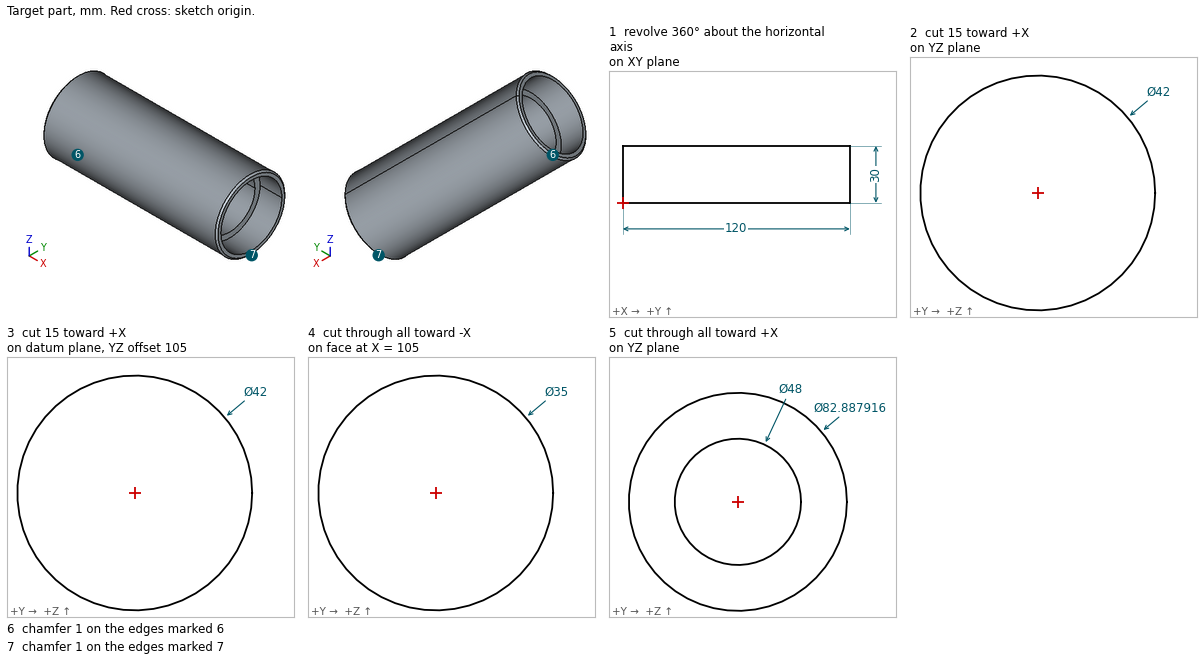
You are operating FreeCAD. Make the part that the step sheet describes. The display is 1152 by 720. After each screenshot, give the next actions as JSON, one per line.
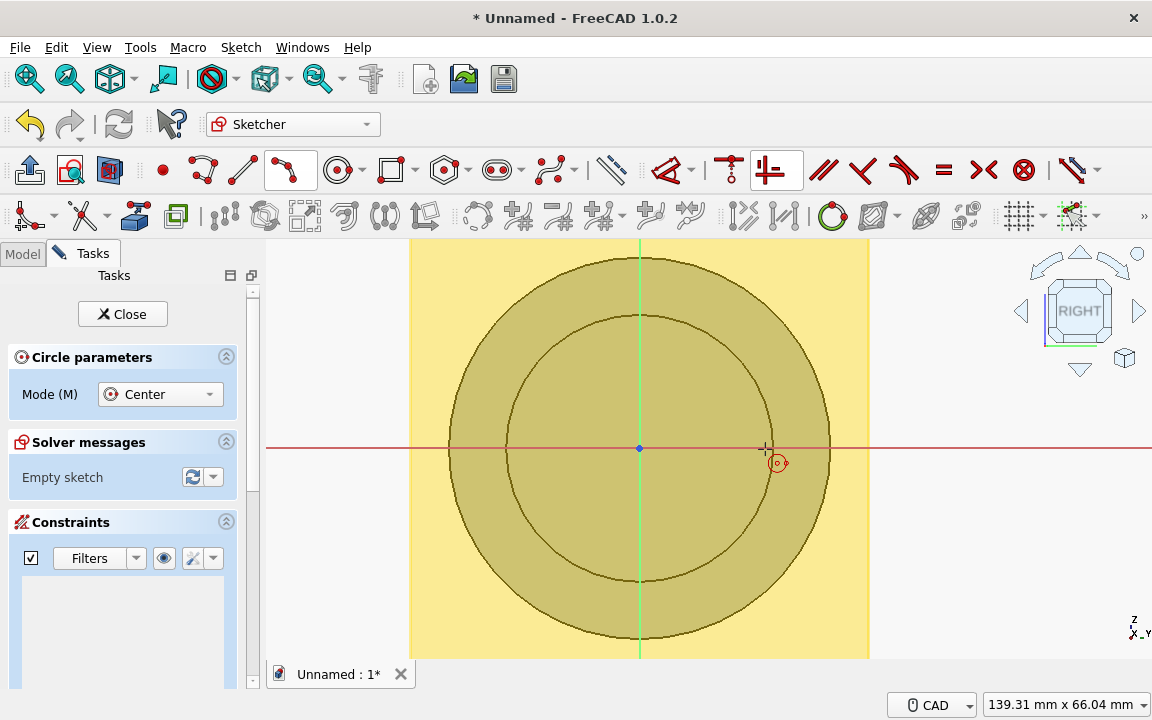
{"action": "left_click", "coordinate": [640, 448]}
{"action": "left_click", "coordinate": [734, 354]}
{"action": "key", "text": "Escape"}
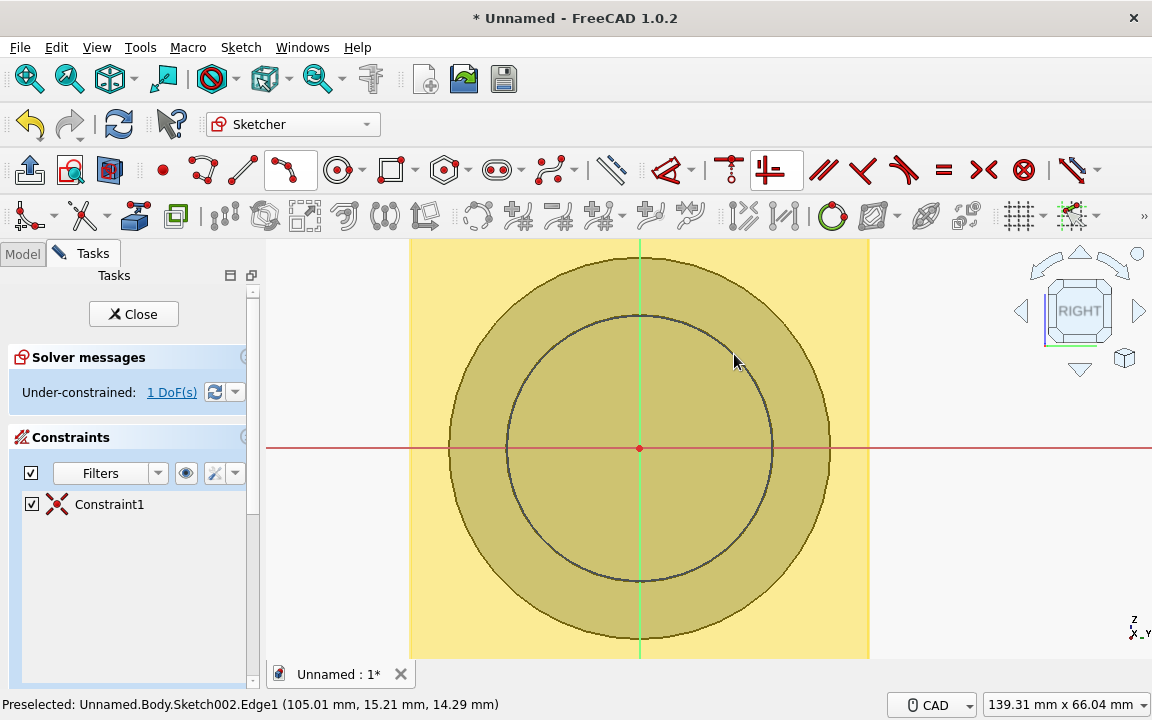
{"action": "key", "text": "d"}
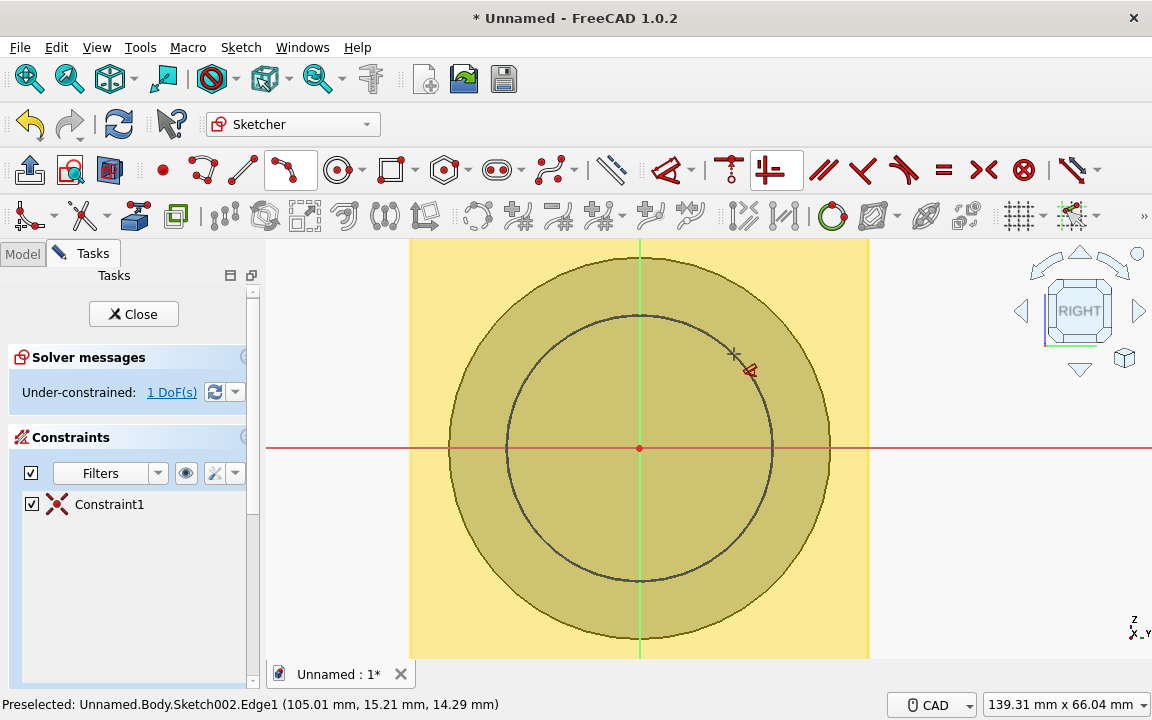
{"action": "left_click", "coordinate": [733, 354]}
{"action": "left_click", "coordinate": [755, 331]}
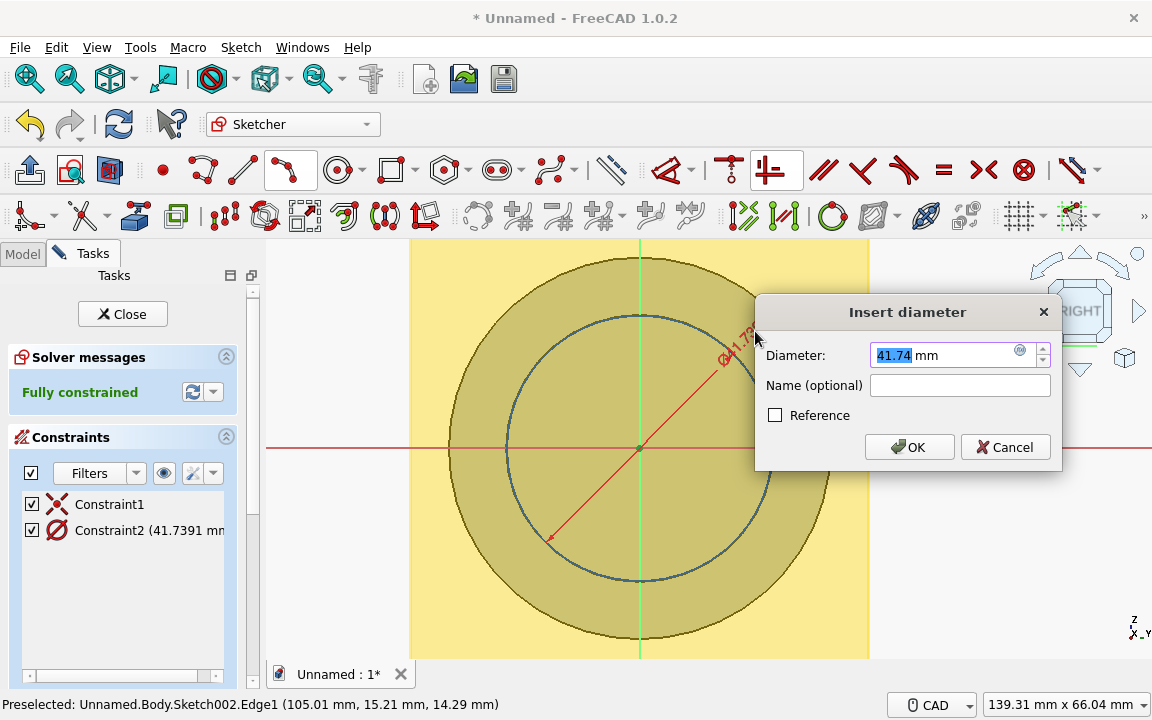
{"action": "type", "text": "42"}
{"action": "key", "text": "Return"}
{"action": "key", "text": "Escape"}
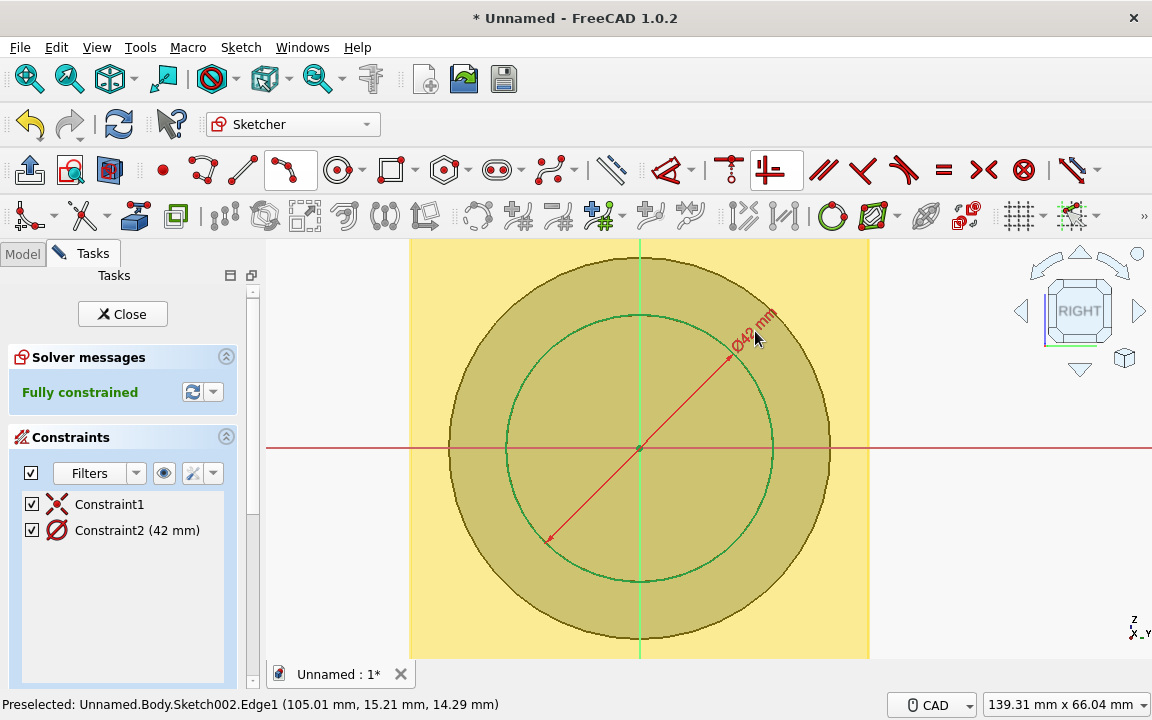
{"action": "left_click", "coordinate": [123, 314]}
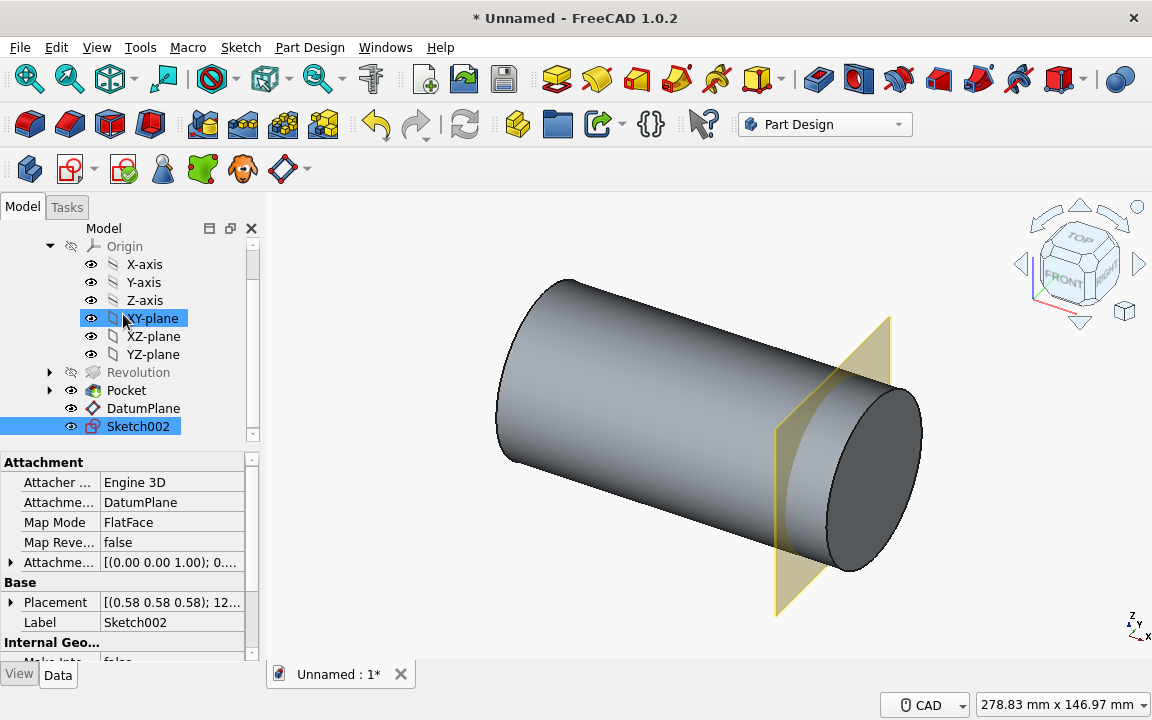
{"action": "left_click", "coordinate": [820, 80]}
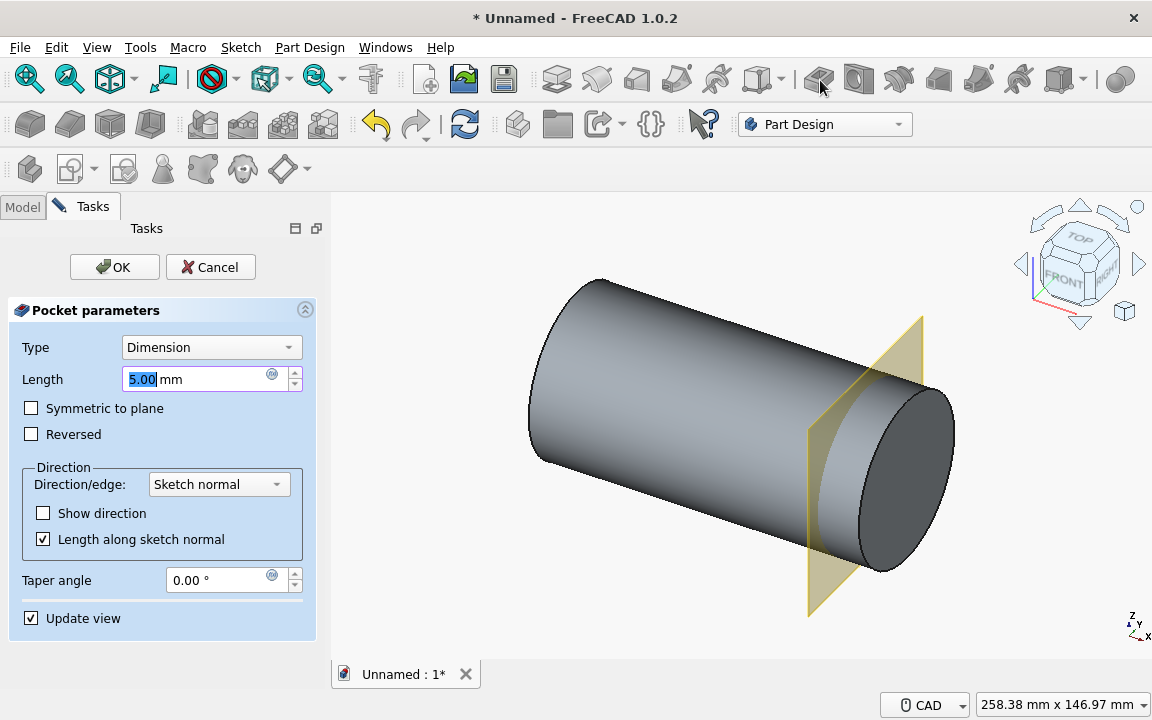
{"action": "type", "text": "15"}
{"action": "key", "text": "Tab"}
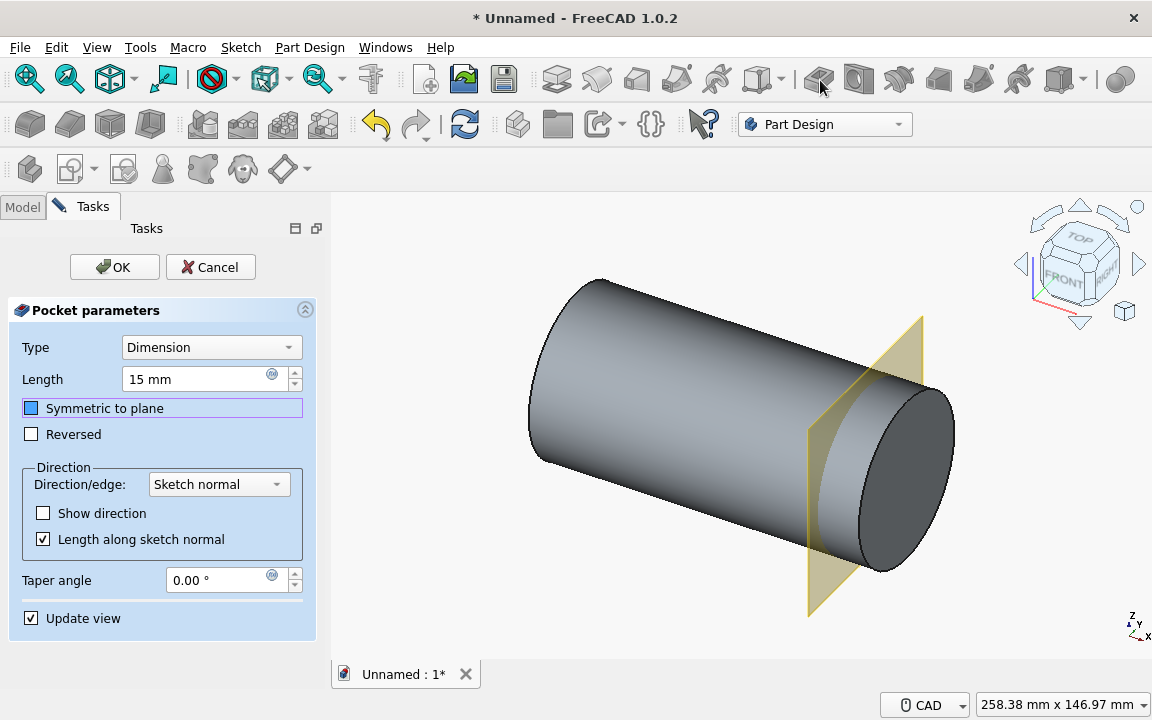
{"action": "left_click", "coordinate": [30, 434]}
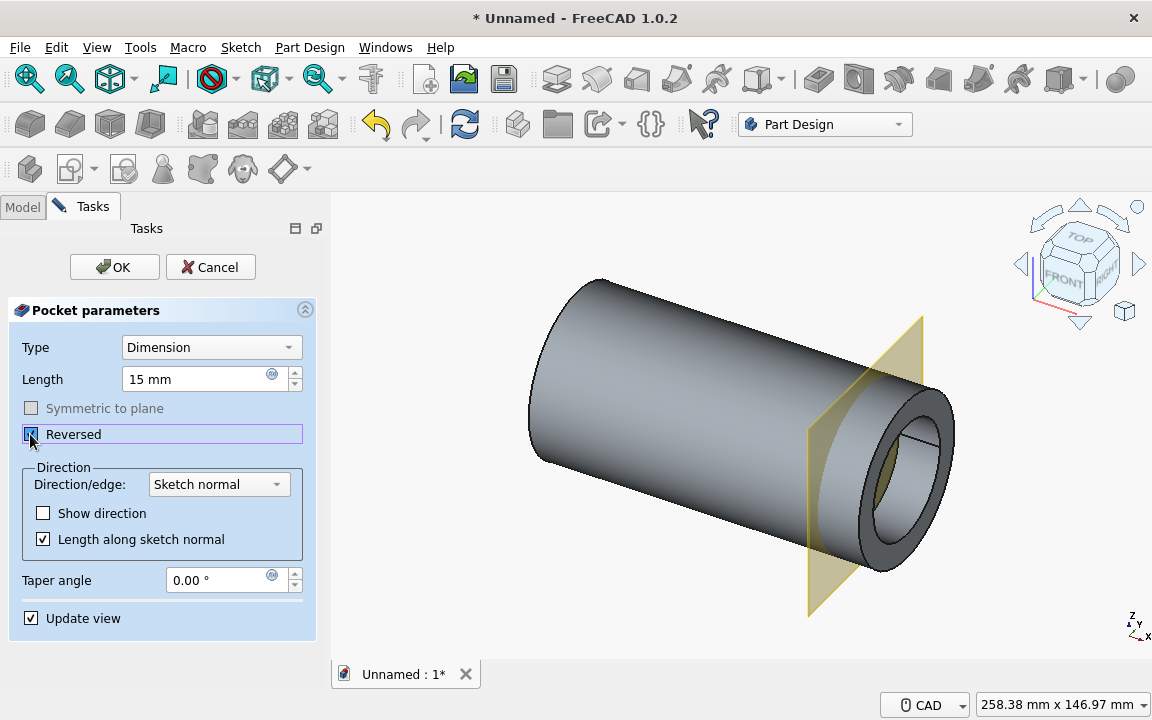
{"action": "left_click", "coordinate": [115, 267]}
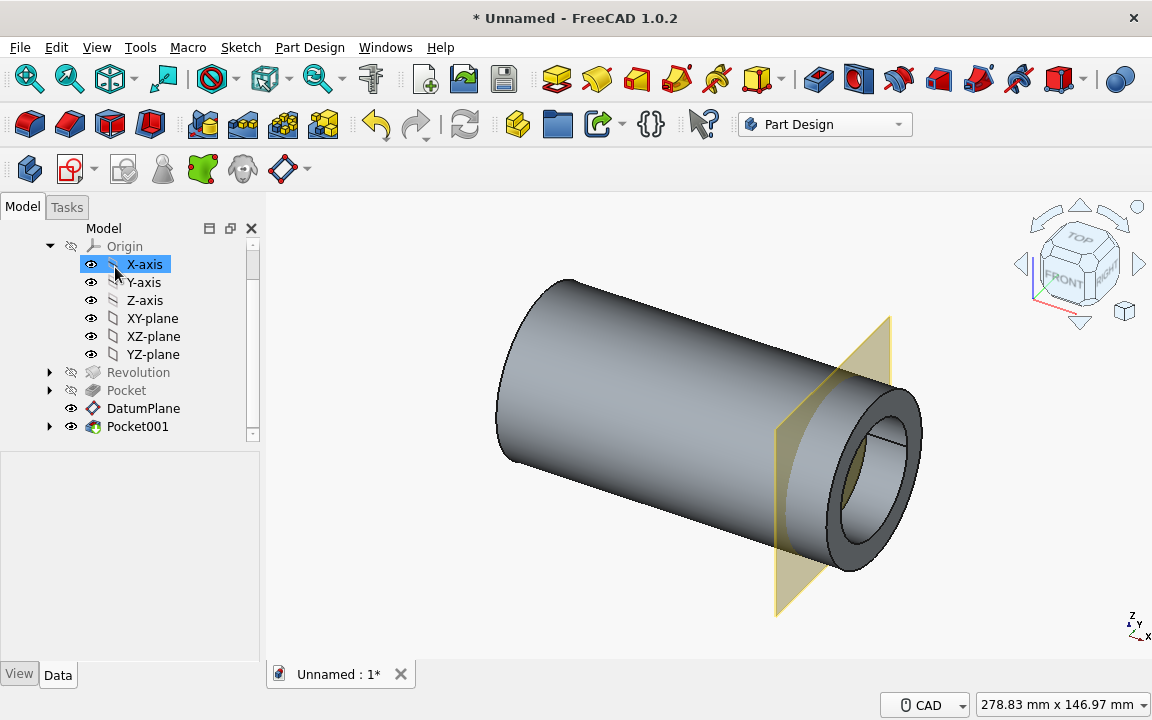
{"action": "left_click", "coordinate": [116, 408]}
{"action": "key", "text": "space"}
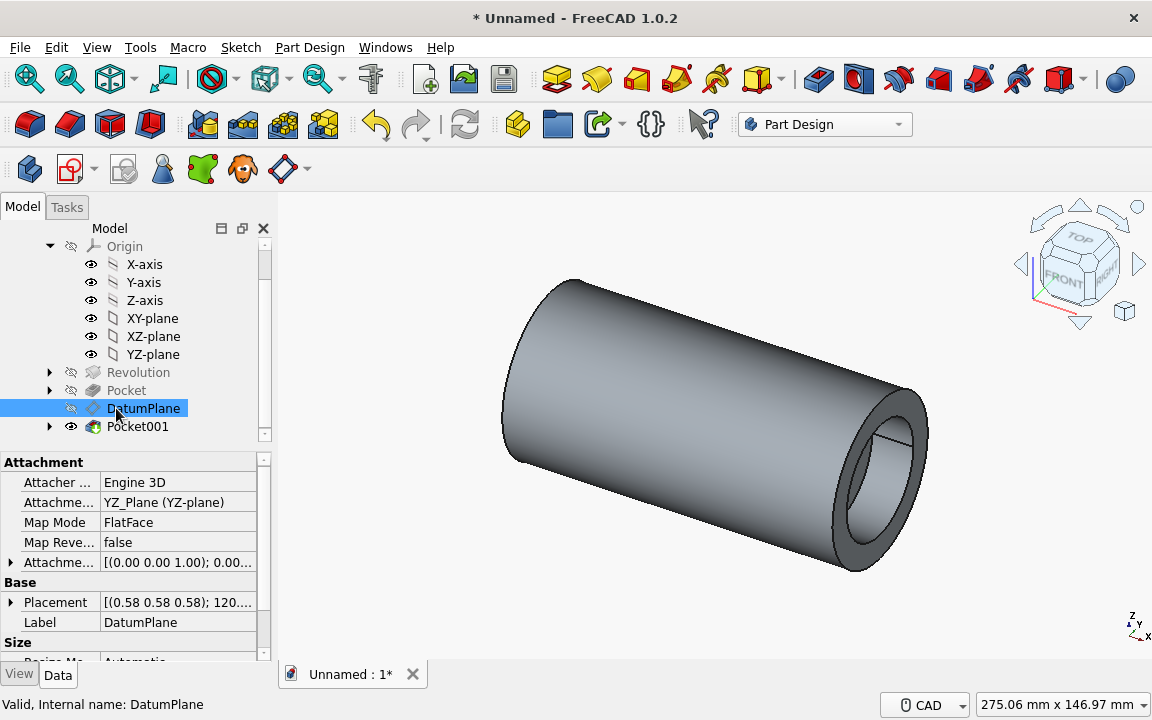
{"action": "key", "text": "0"}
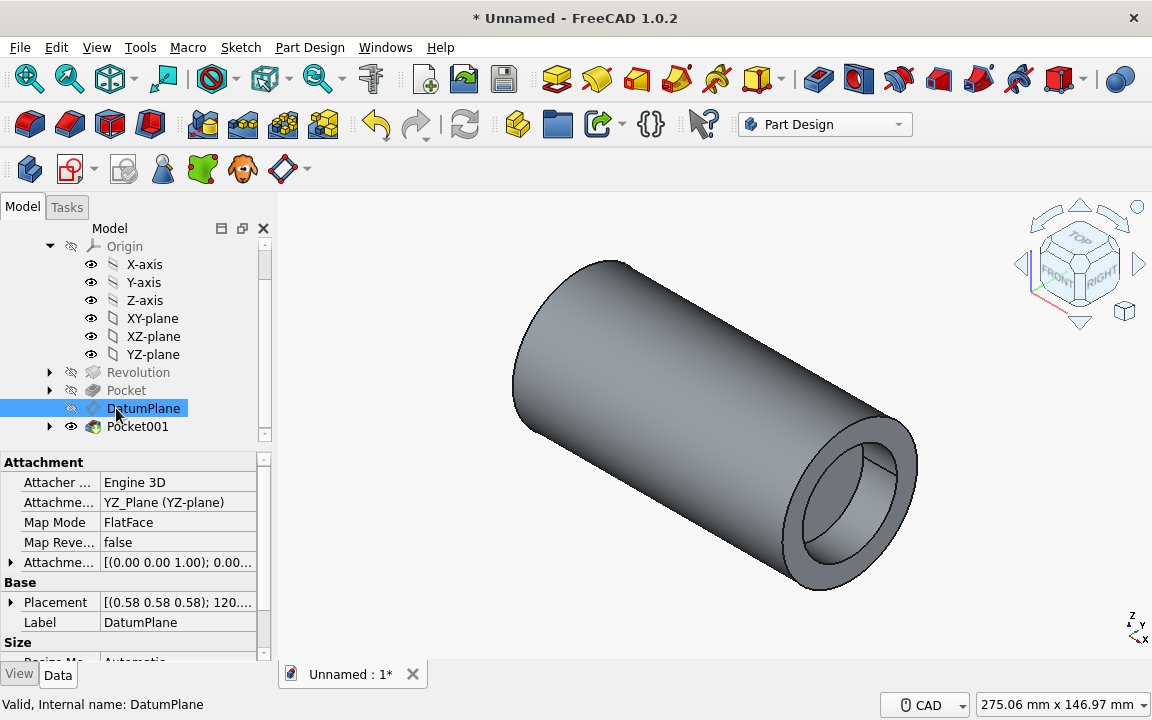
{"action": "left_click", "coordinate": [830, 491]}